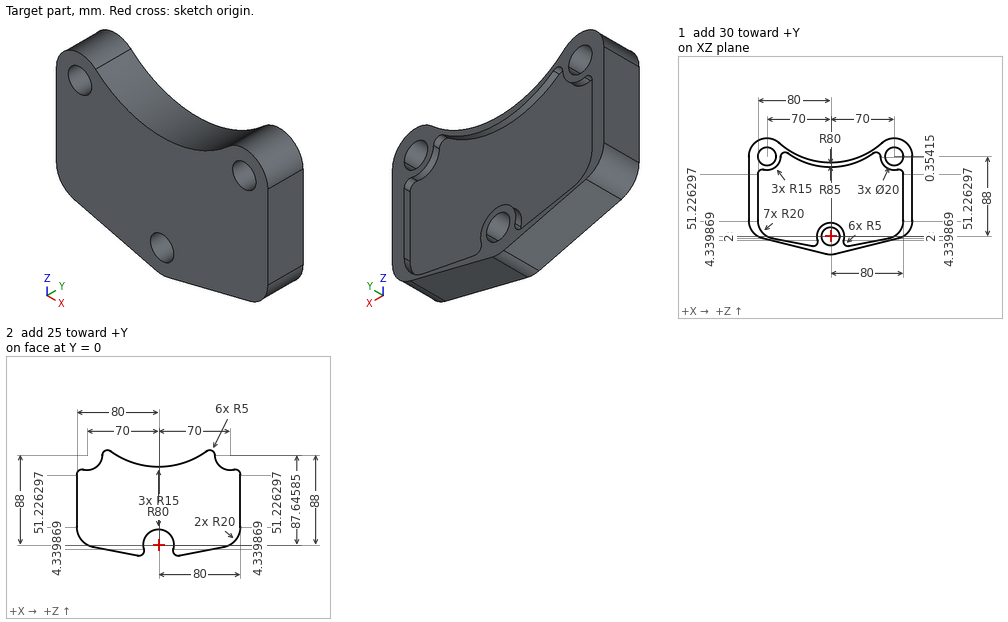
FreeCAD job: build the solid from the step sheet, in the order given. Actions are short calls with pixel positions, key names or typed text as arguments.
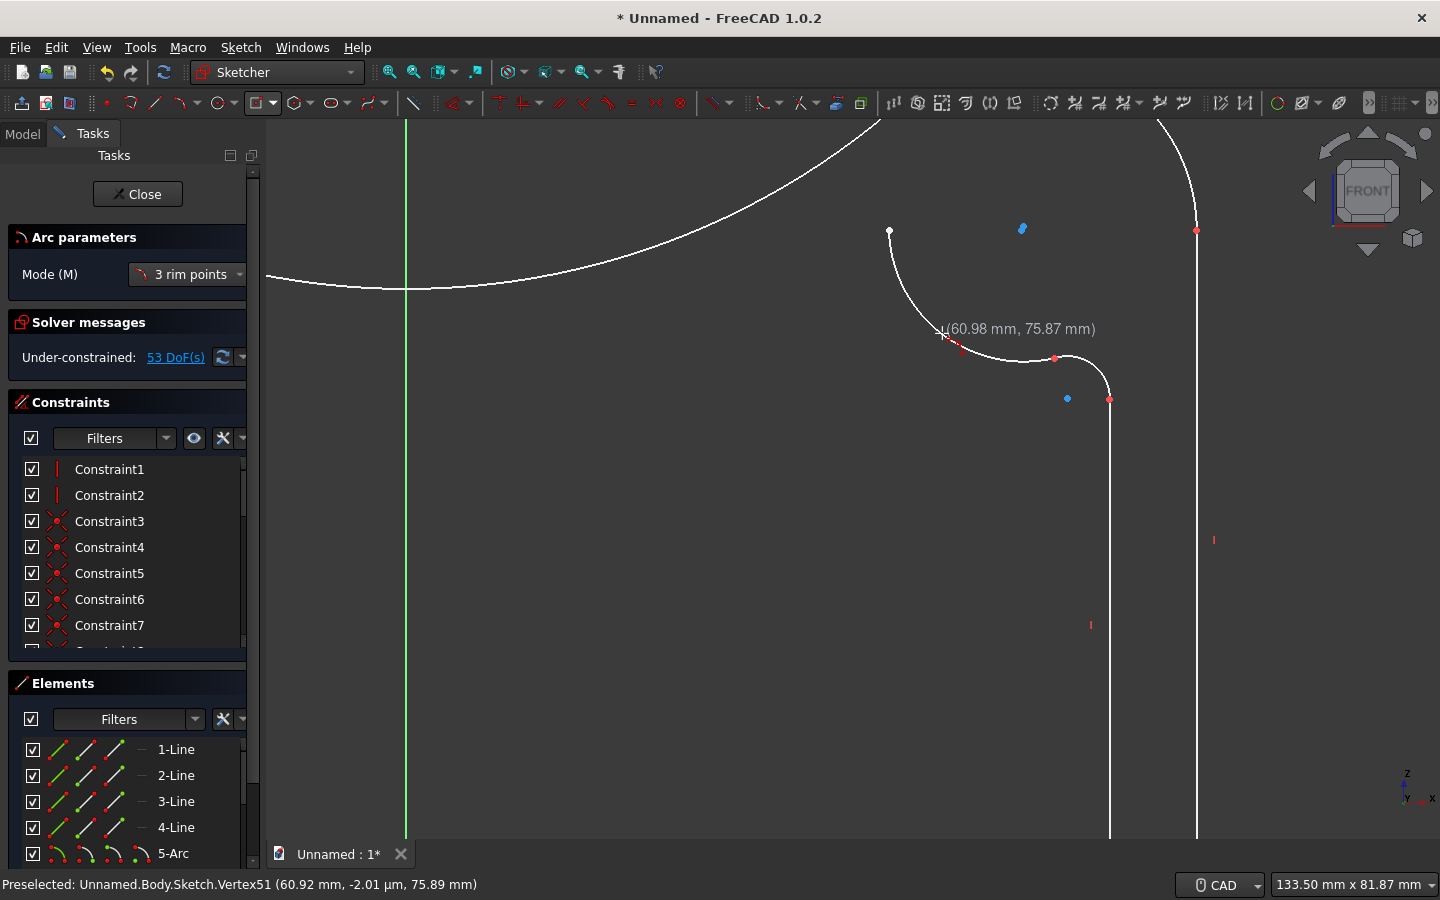
click(889, 231)
click(820, 196)
click(865, 192)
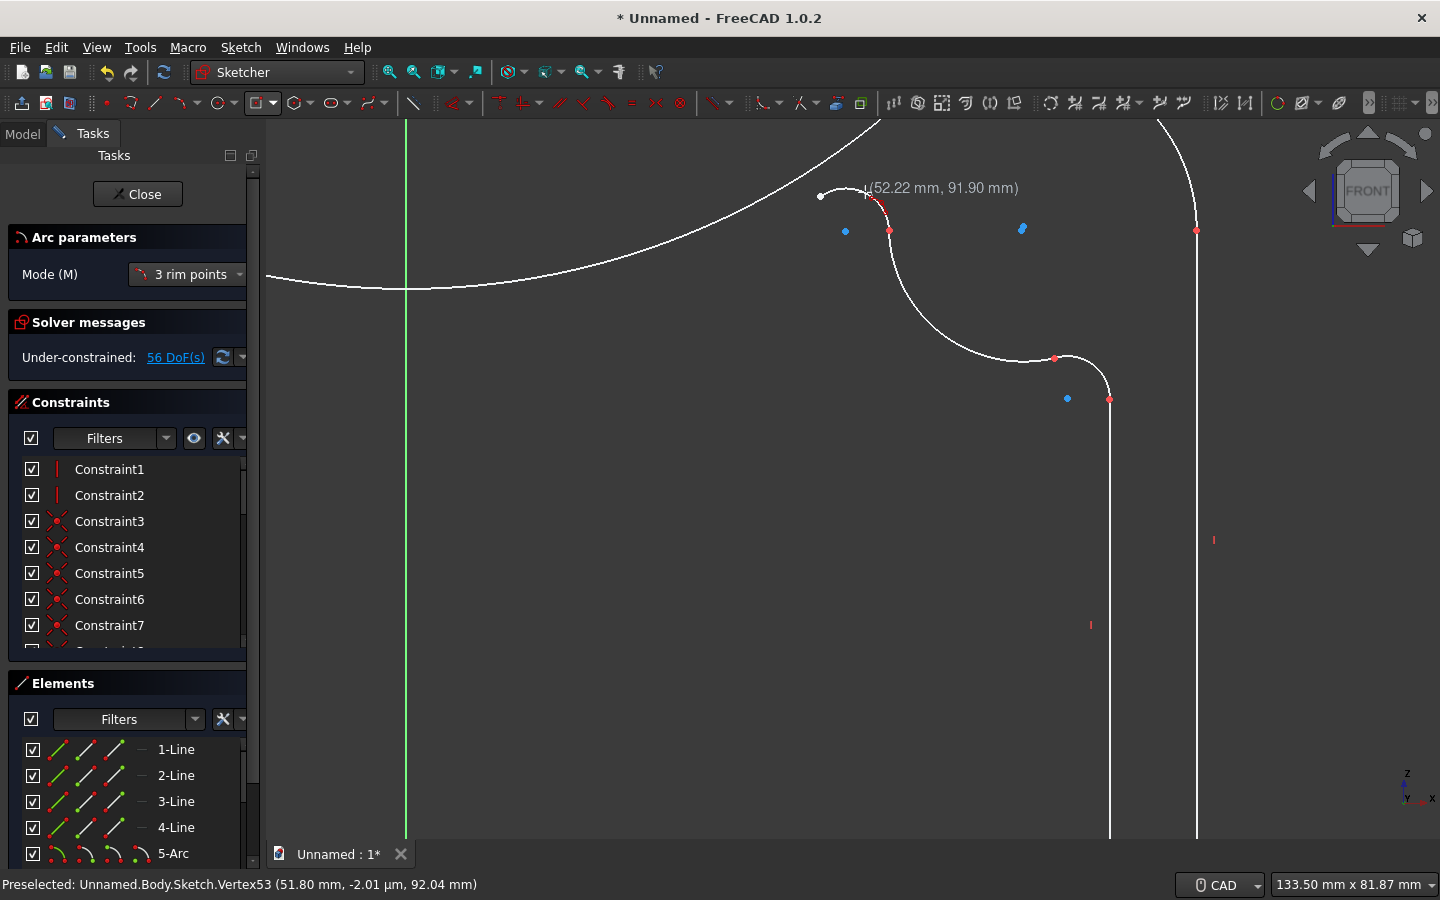
click(820, 197)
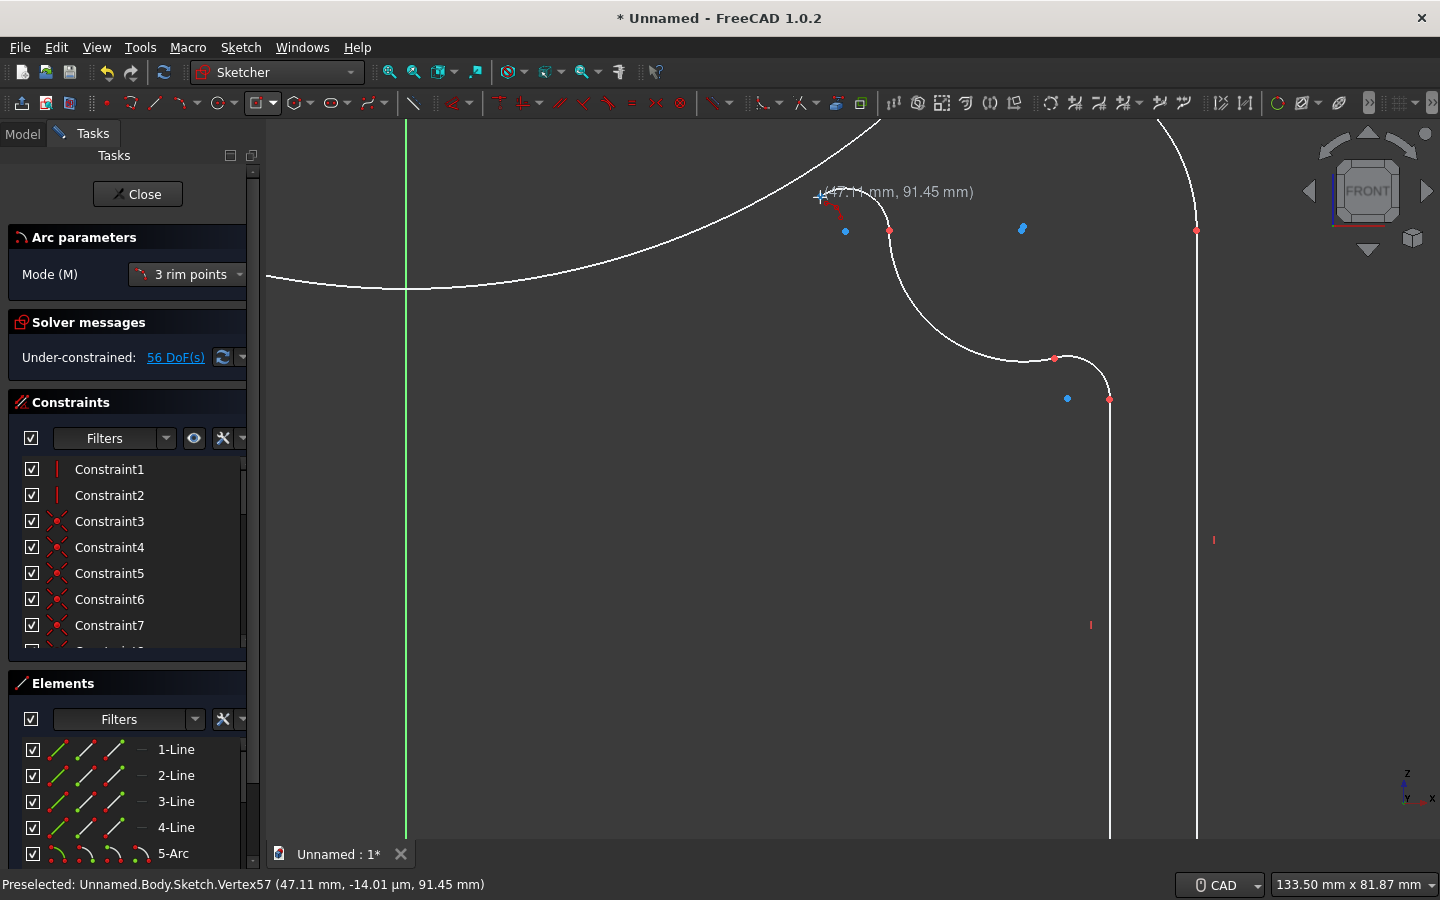
scroll(1094, 362, down, 4)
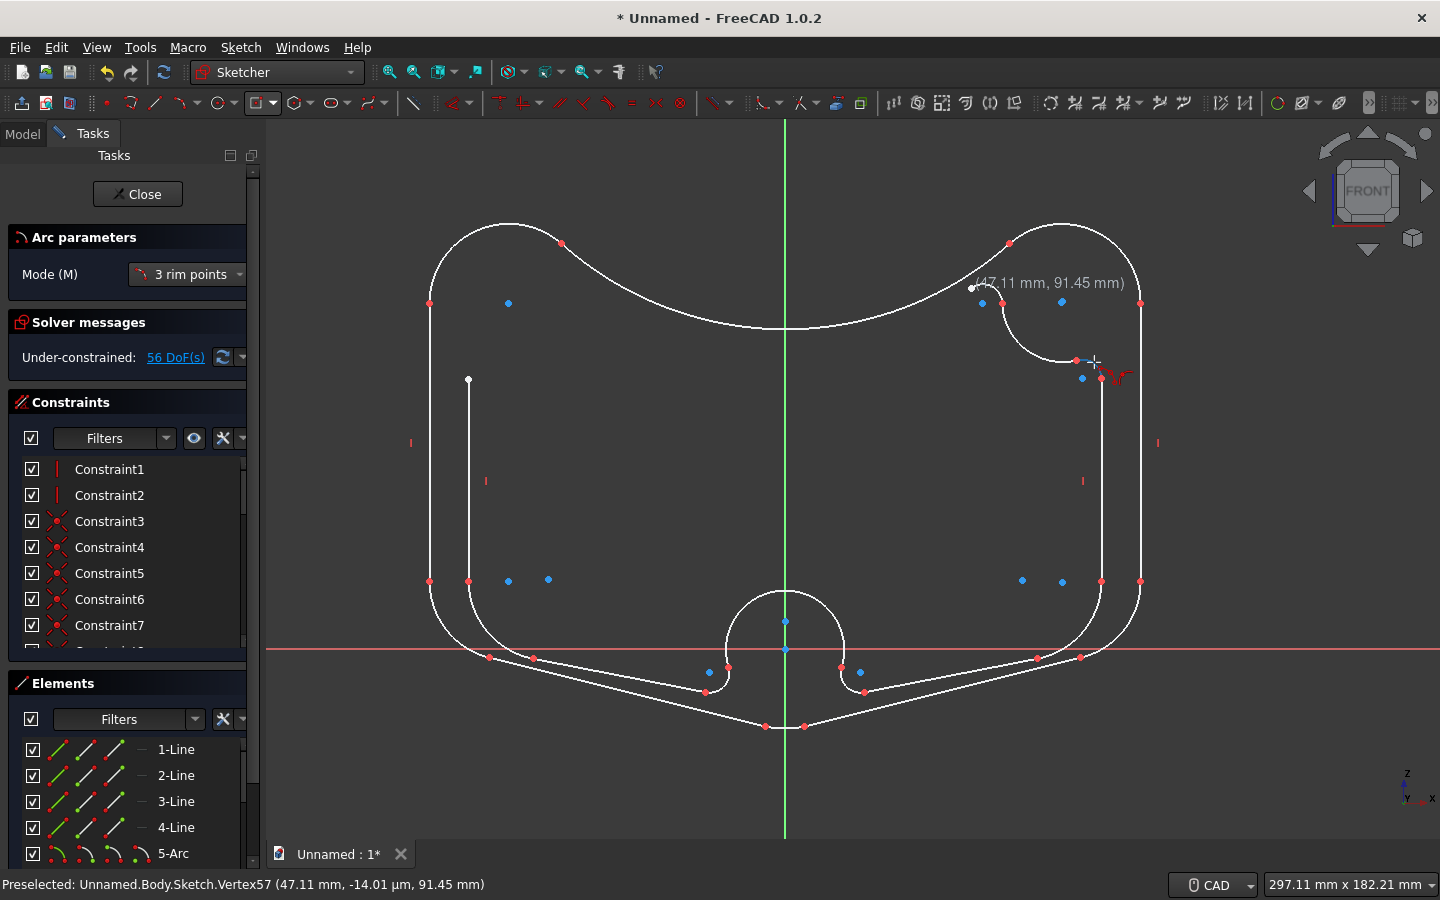
scroll(599, 288, up, 2)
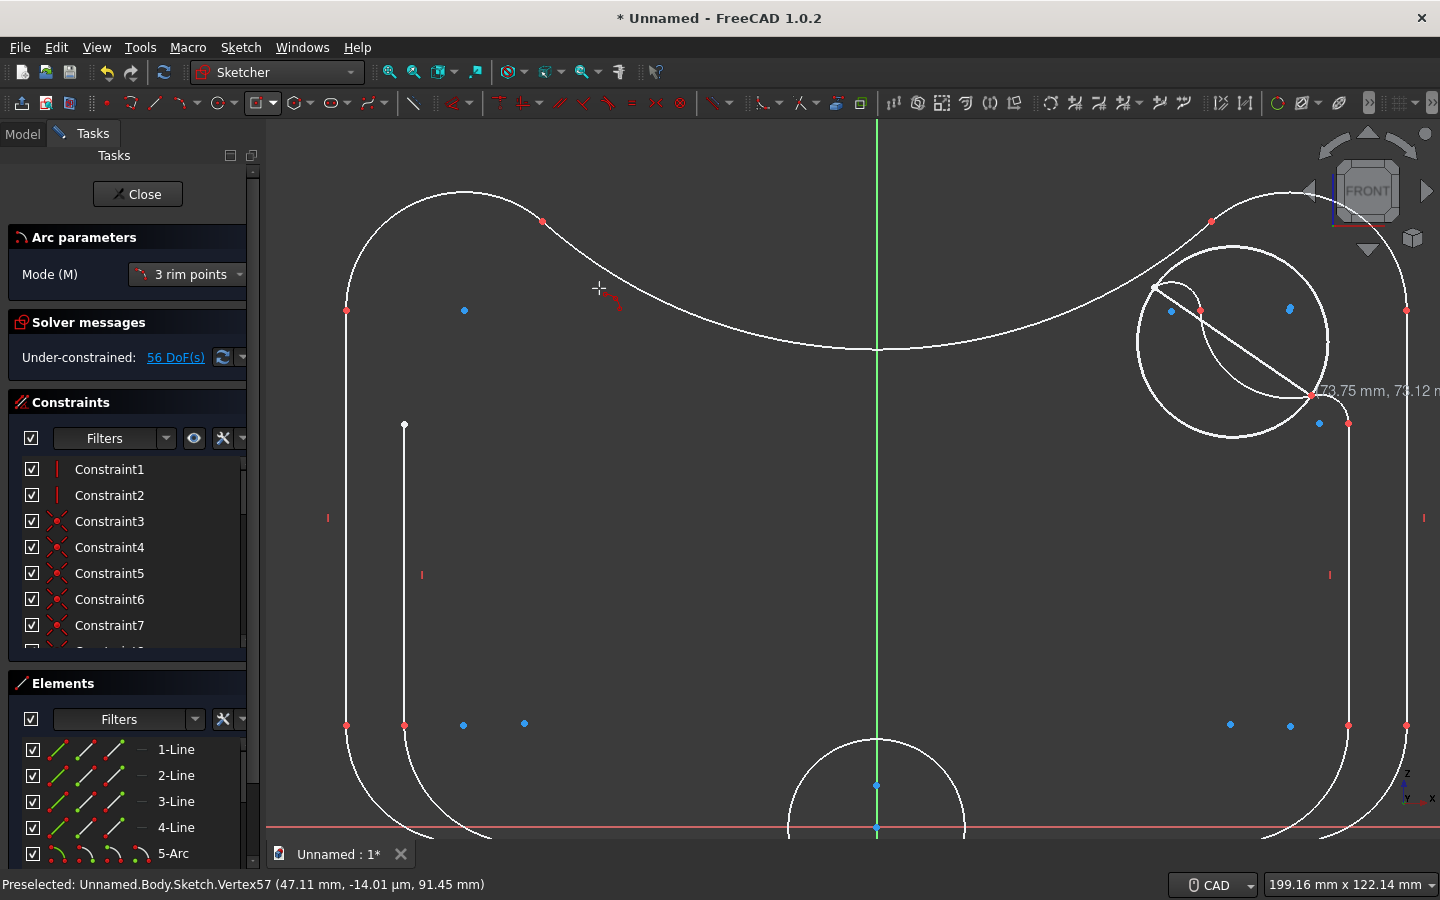
click(599, 287)
click(817, 374)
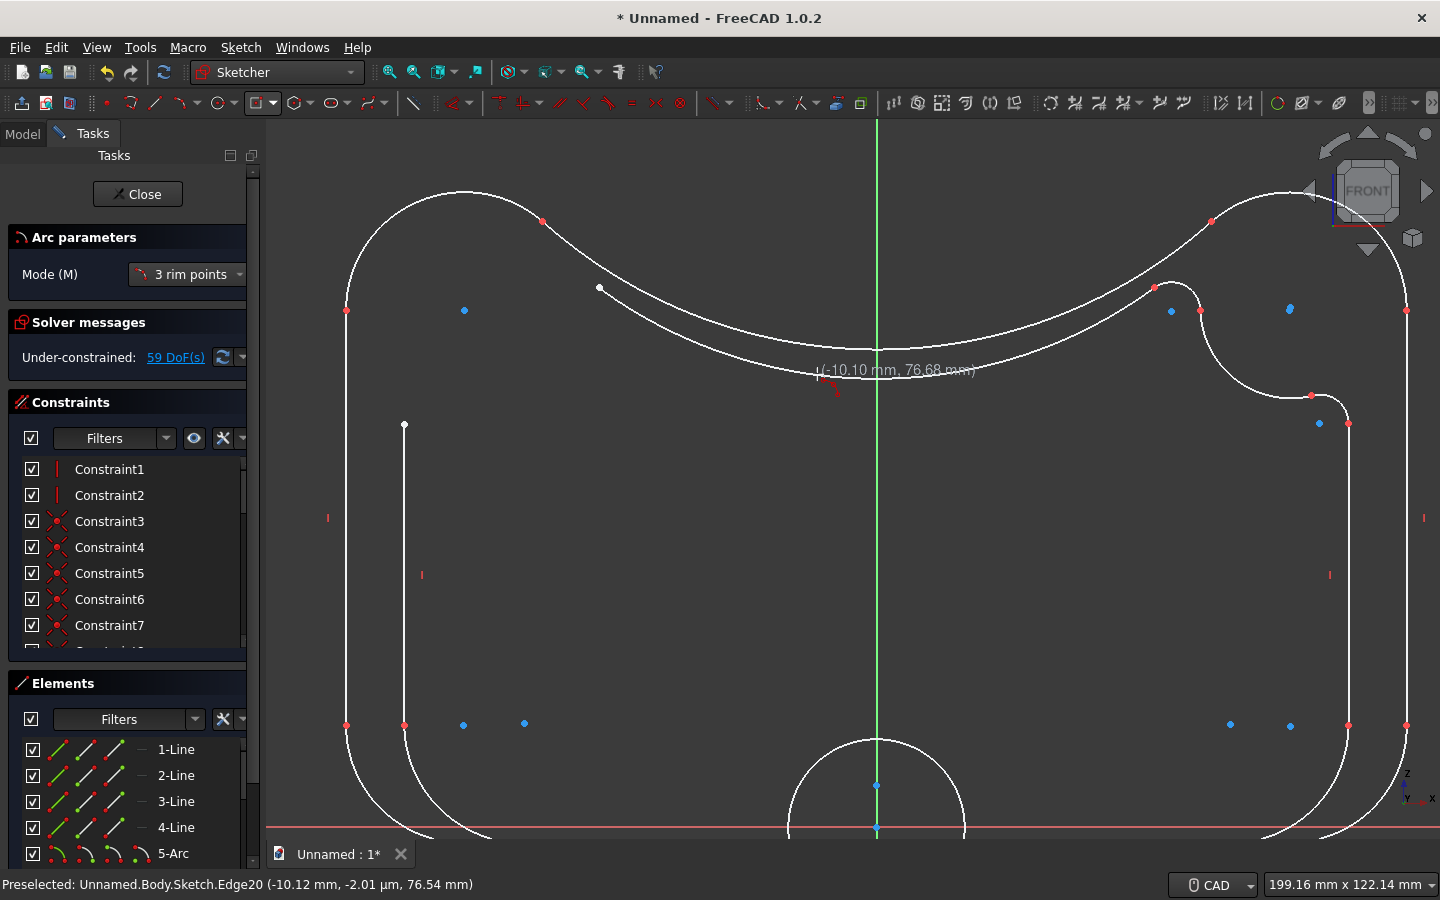
click(599, 288)
click(552, 310)
click(569, 285)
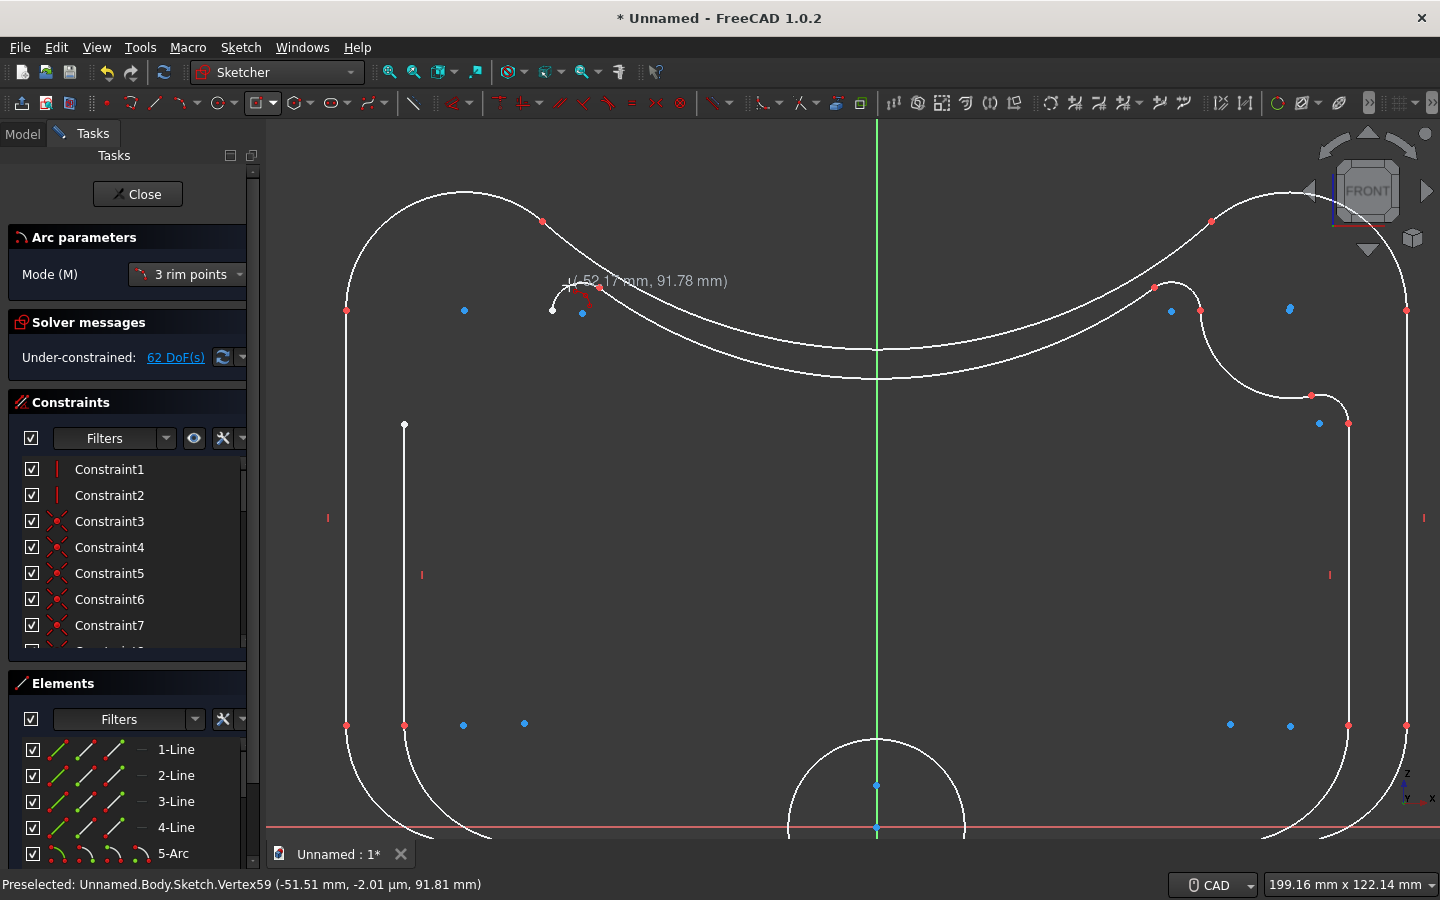
click(552, 311)
click(442, 394)
click(517, 379)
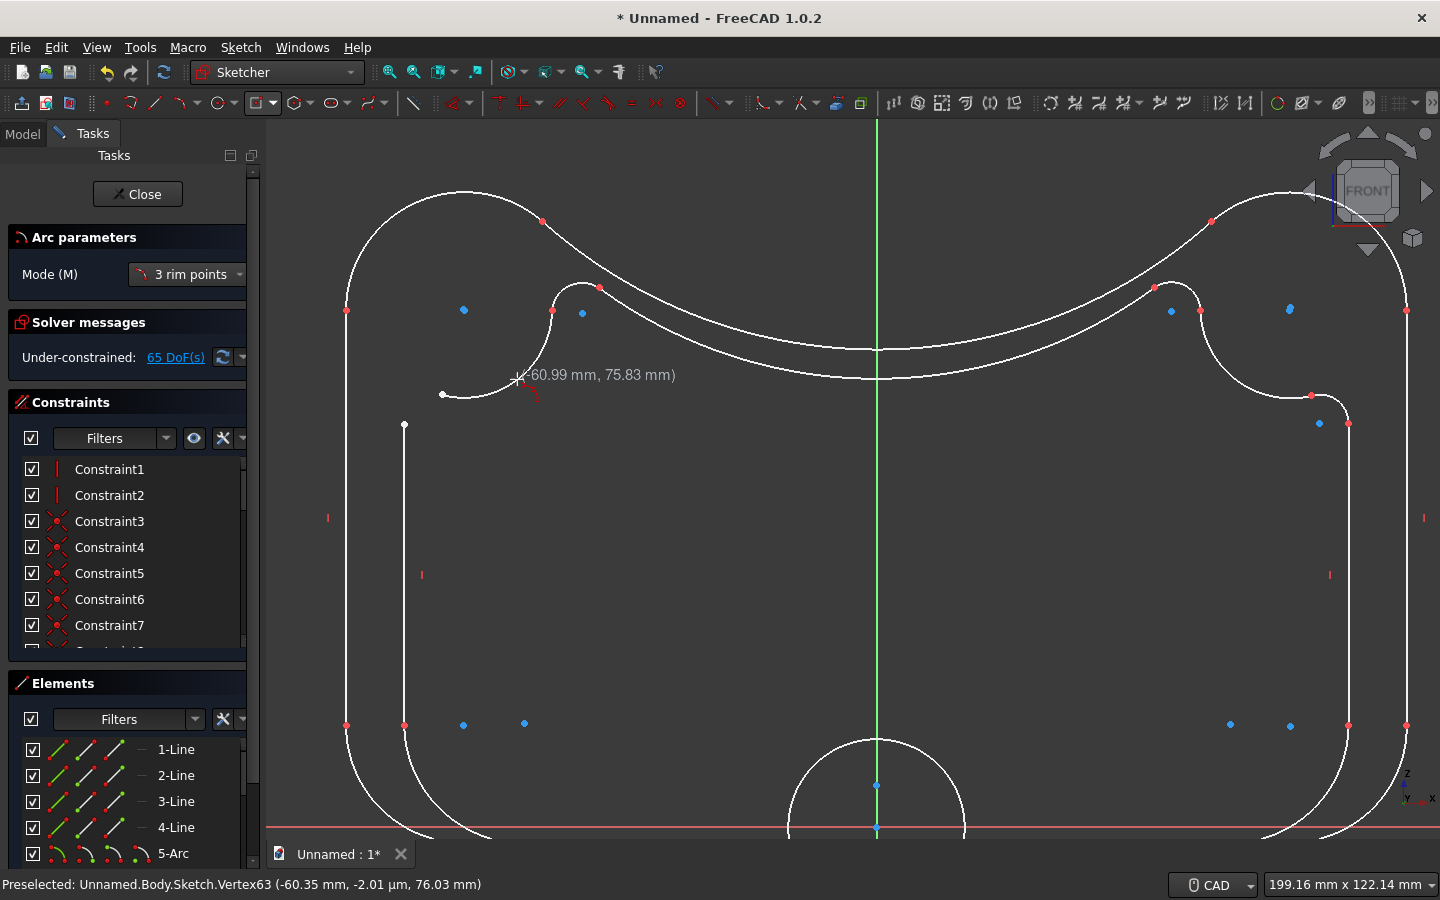
click(442, 395)
click(404, 424)